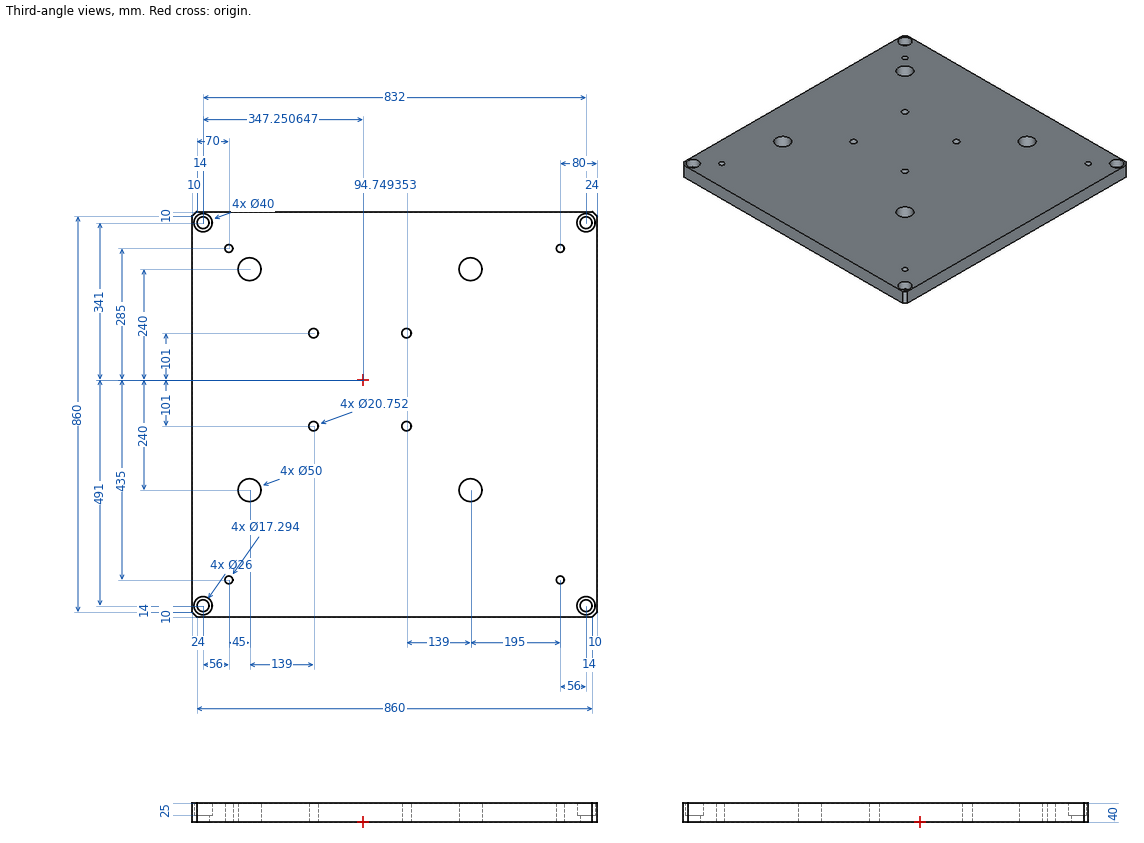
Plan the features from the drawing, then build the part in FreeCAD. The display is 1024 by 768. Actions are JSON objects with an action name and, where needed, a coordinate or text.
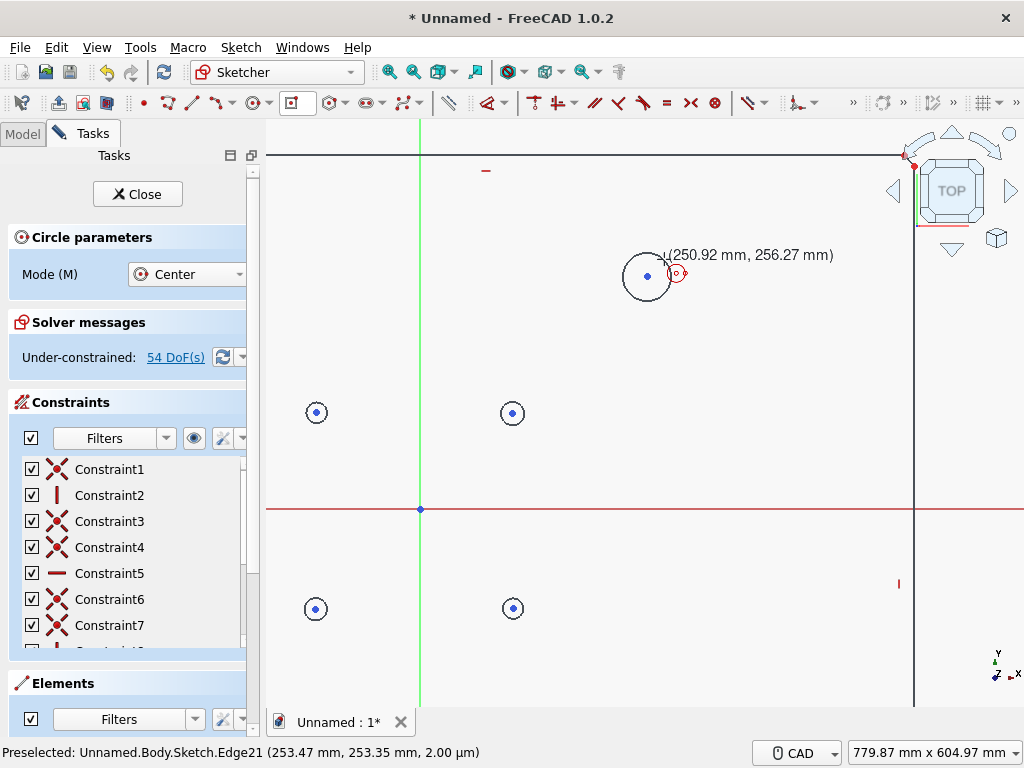
{"action": "scroll", "coordinate": [837, 232], "scroll_direction": "up", "scroll_amount": 5}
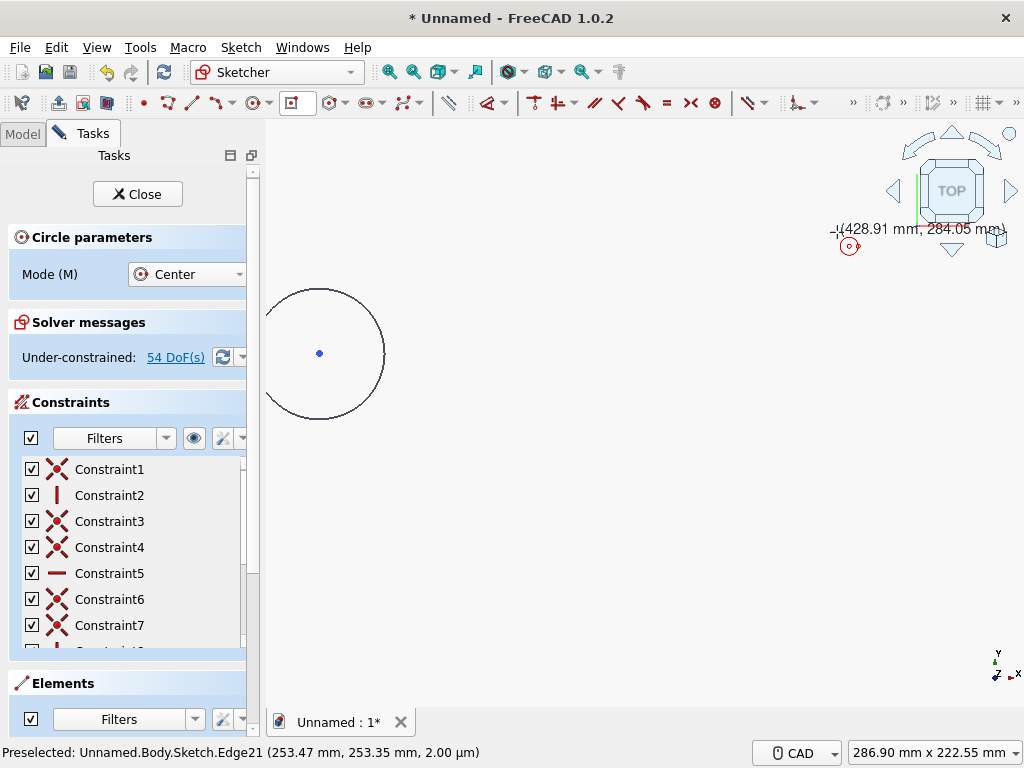
{"action": "scroll", "coordinate": [714, 261], "scroll_direction": "down", "scroll_amount": 9}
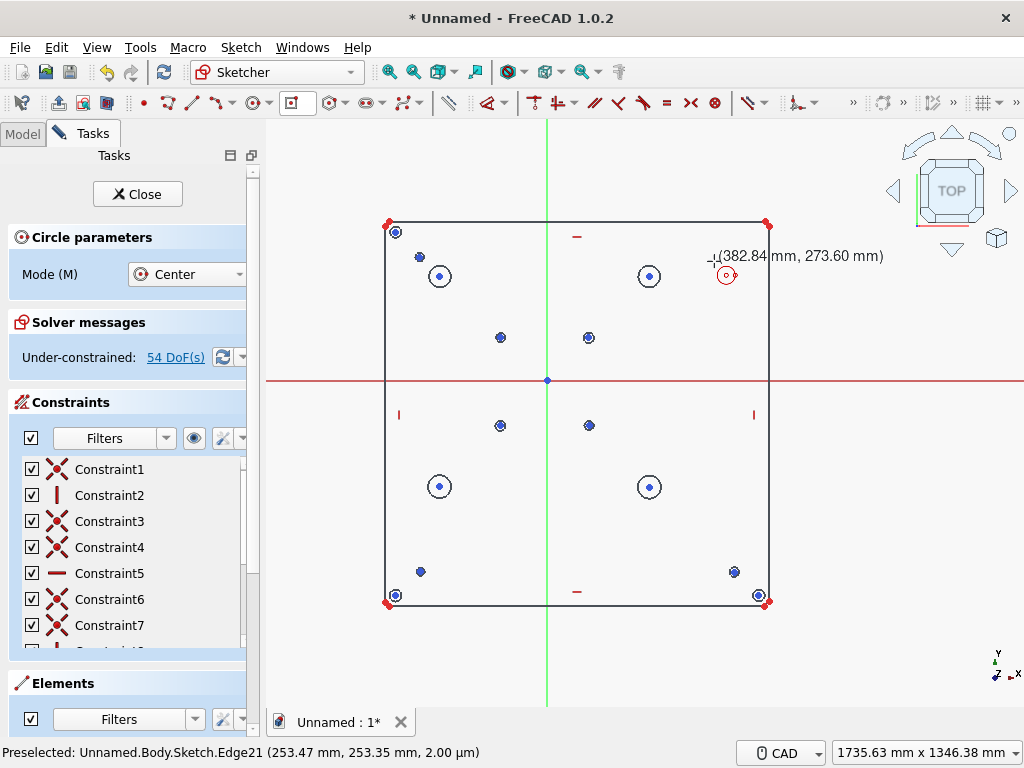
{"action": "left_click", "coordinate": [735, 256]}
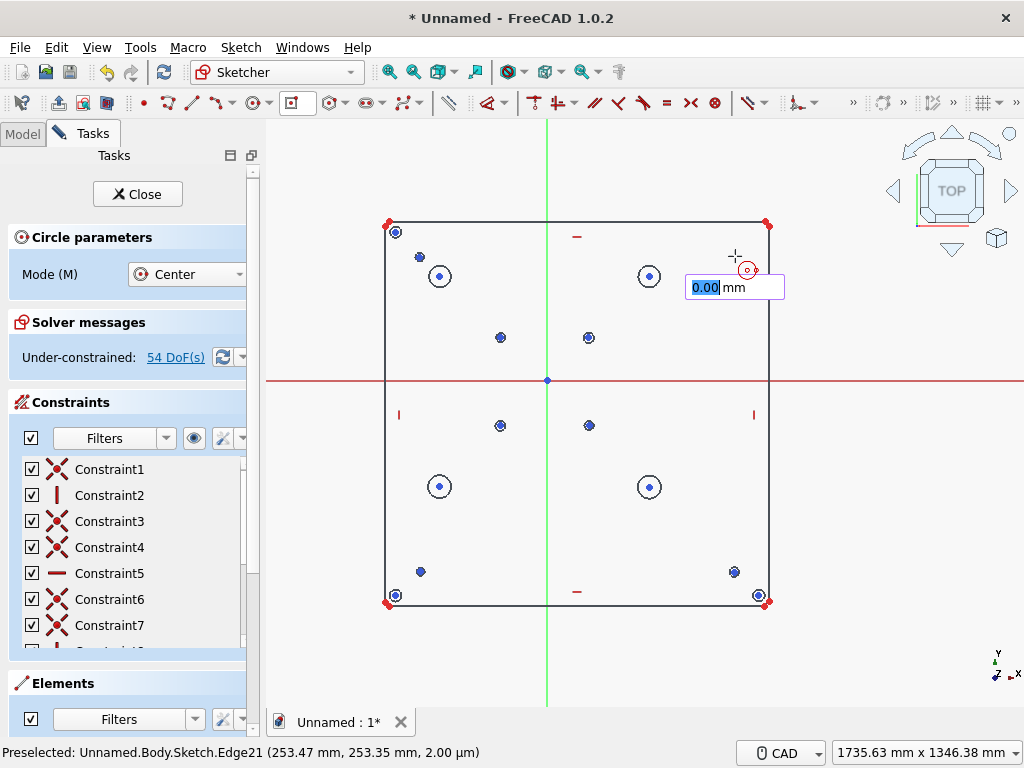
{"action": "scroll", "coordinate": [737, 254], "scroll_direction": "up", "scroll_amount": 8}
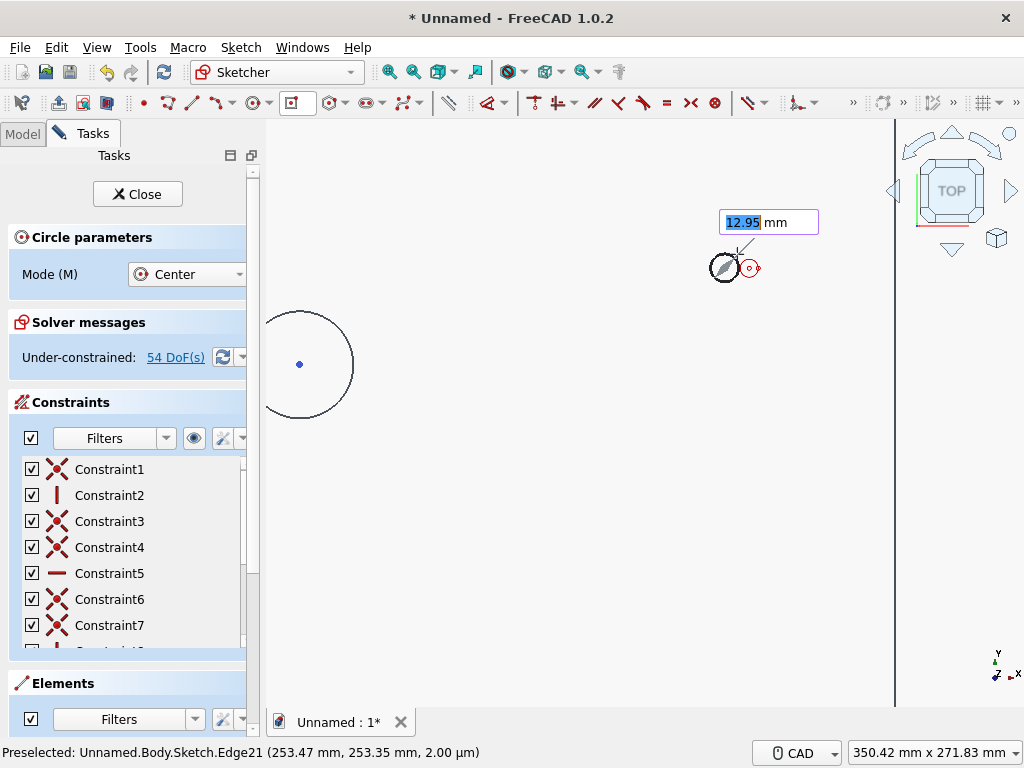
{"action": "left_click", "coordinate": [736, 252]}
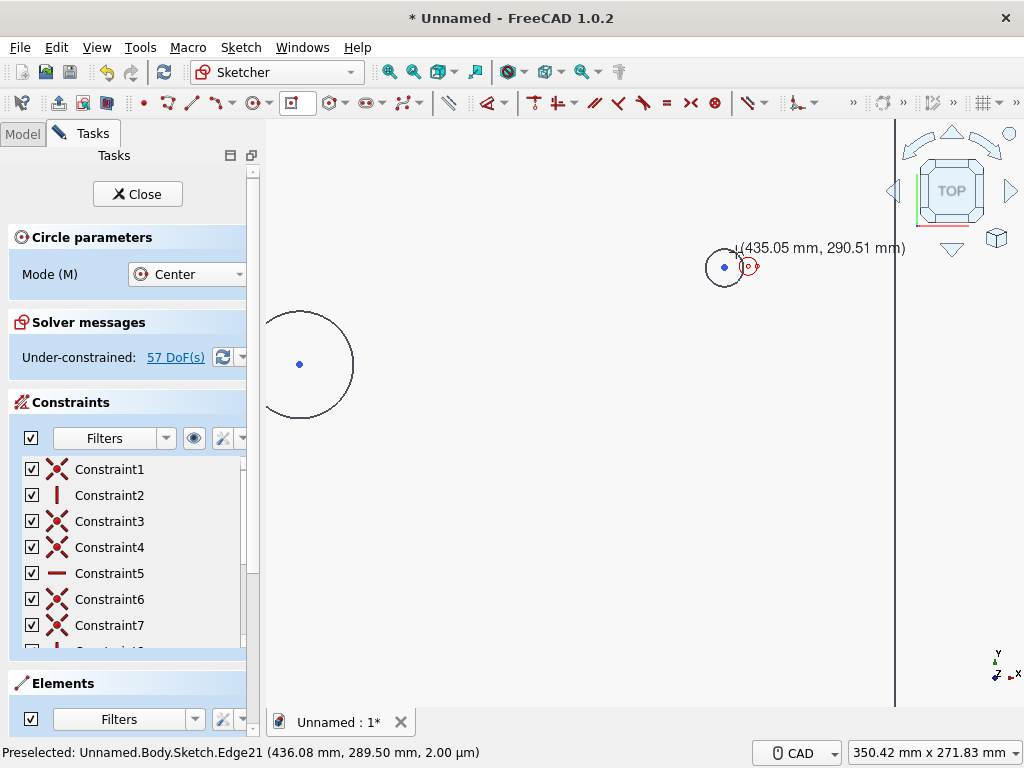
{"action": "scroll", "coordinate": [737, 253], "scroll_direction": "down", "scroll_amount": 8}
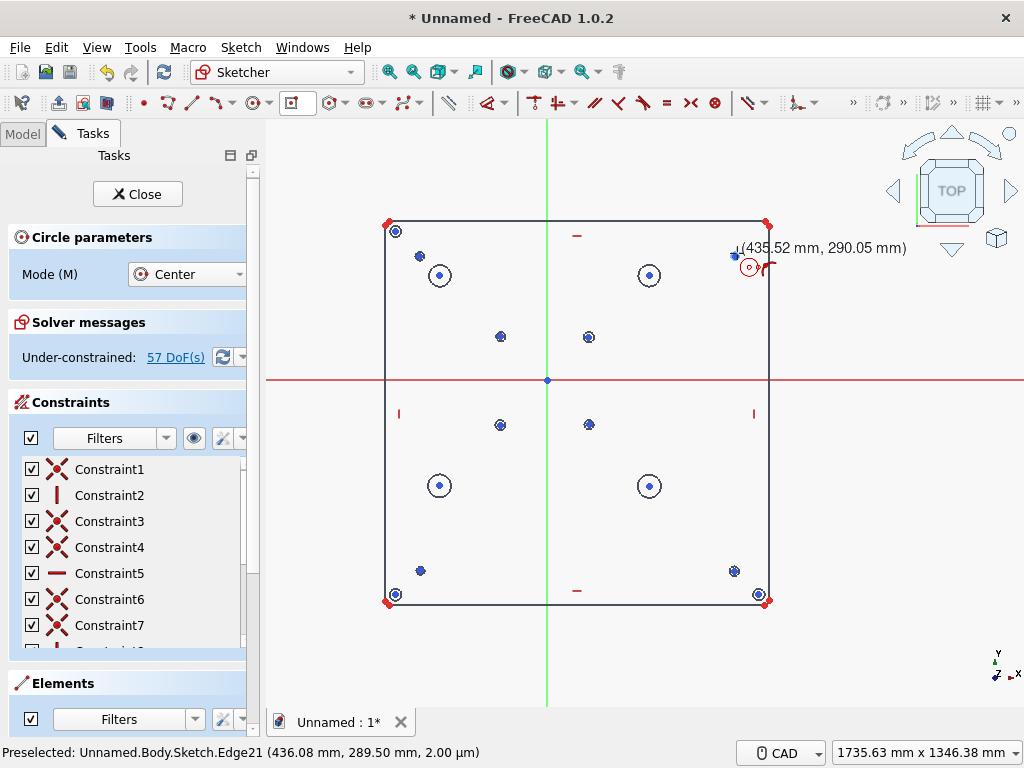
{"action": "scroll", "coordinate": [759, 231], "scroll_direction": "up", "scroll_amount": 7}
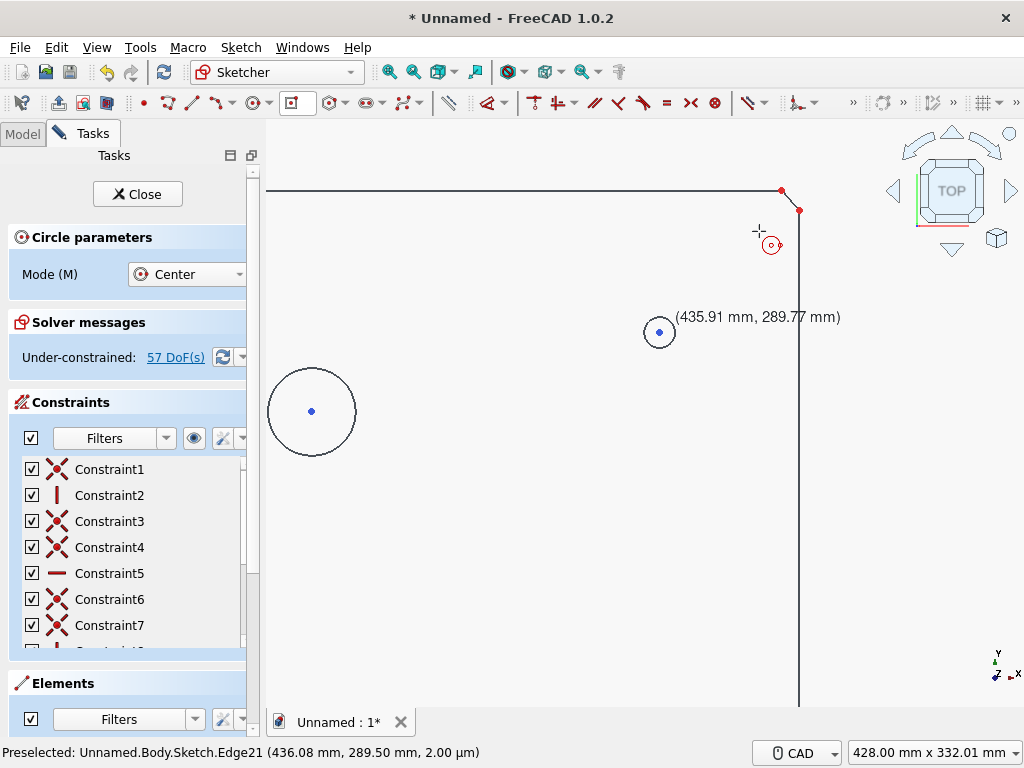
{"action": "left_click", "coordinate": [757, 231]}
{"action": "left_click", "coordinate": [773, 215]}
{"action": "key", "text": "Escape"}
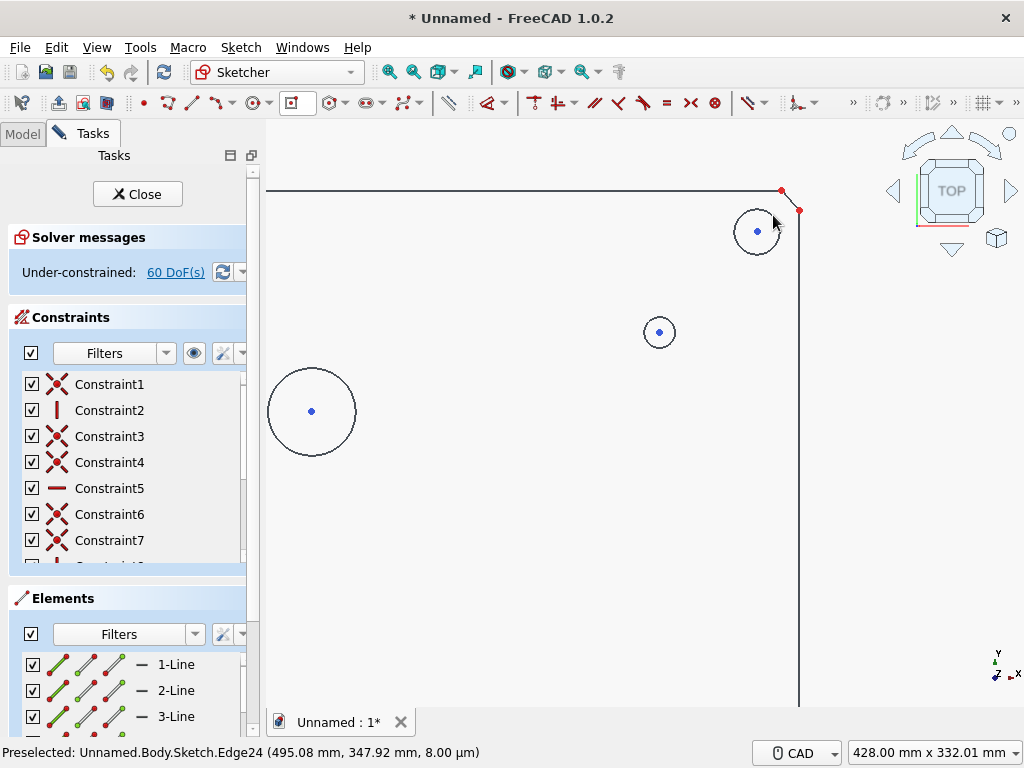
{"action": "scroll", "coordinate": [759, 231], "scroll_direction": "down", "scroll_amount": 7}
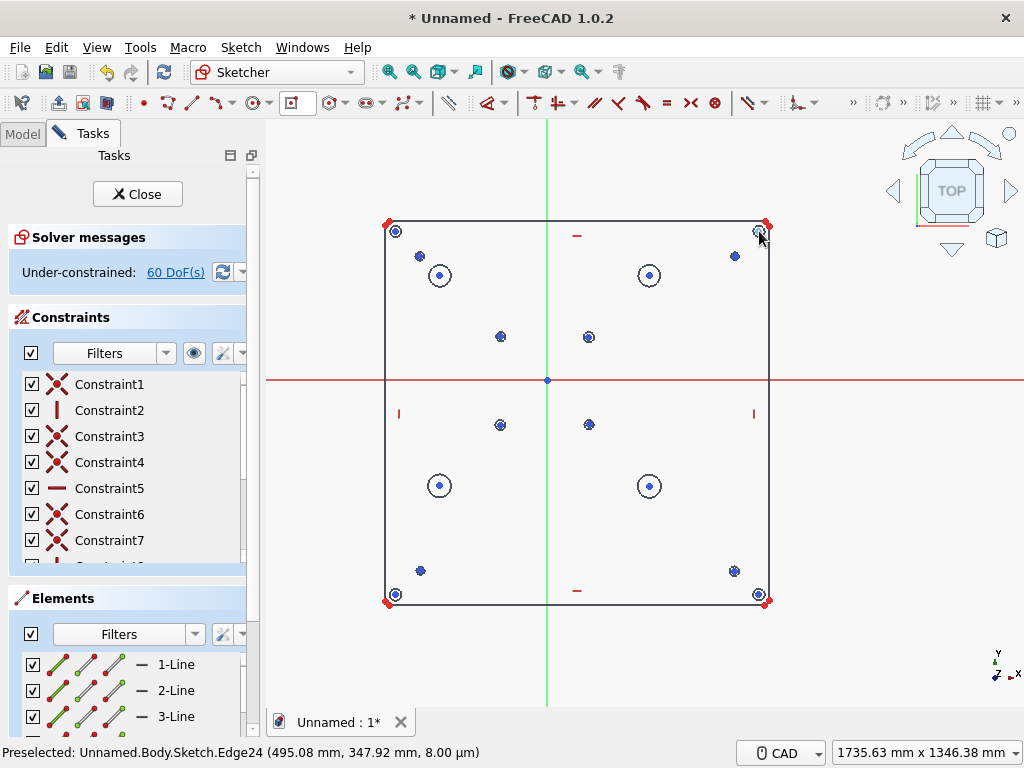
{"action": "scroll", "coordinate": [400, 591], "scroll_direction": "up", "scroll_amount": 5}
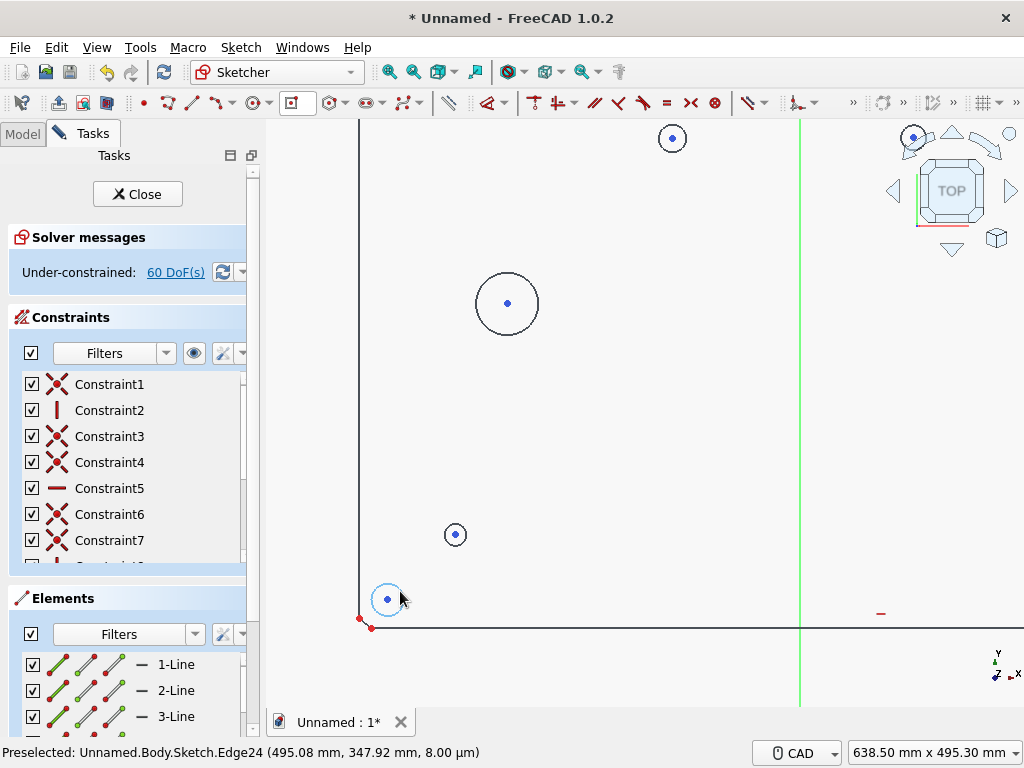
{"action": "left_click", "coordinate": [399, 589]}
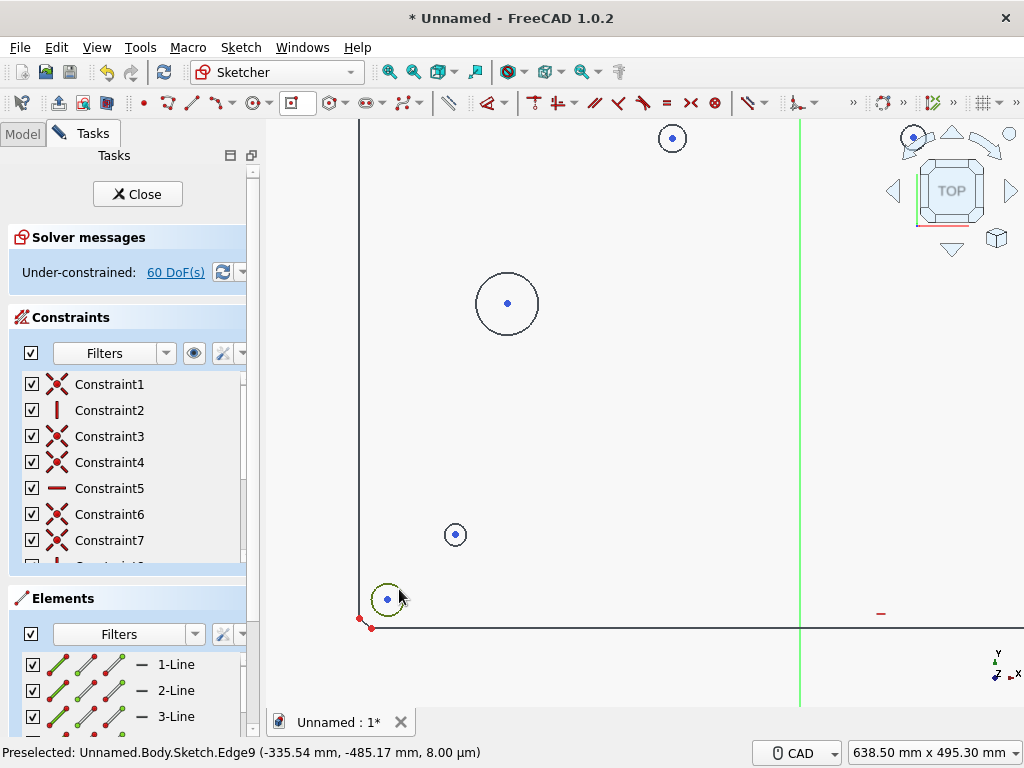
{"action": "scroll", "coordinate": [399, 592], "scroll_direction": "down", "scroll_amount": 5}